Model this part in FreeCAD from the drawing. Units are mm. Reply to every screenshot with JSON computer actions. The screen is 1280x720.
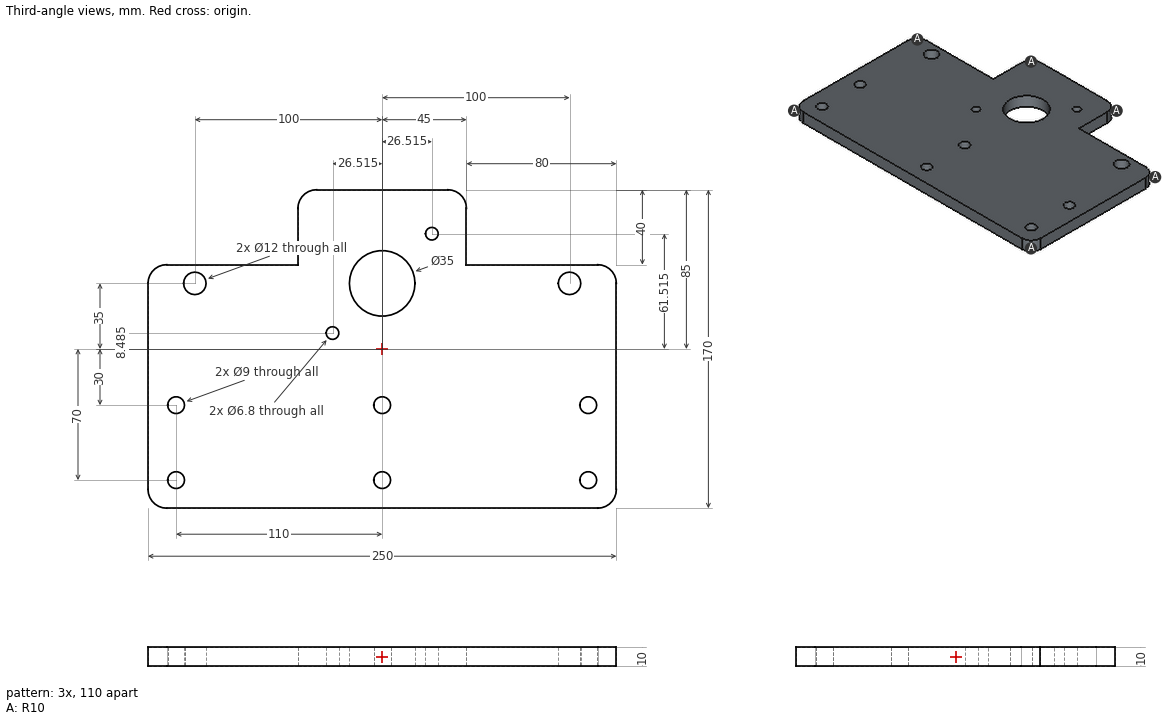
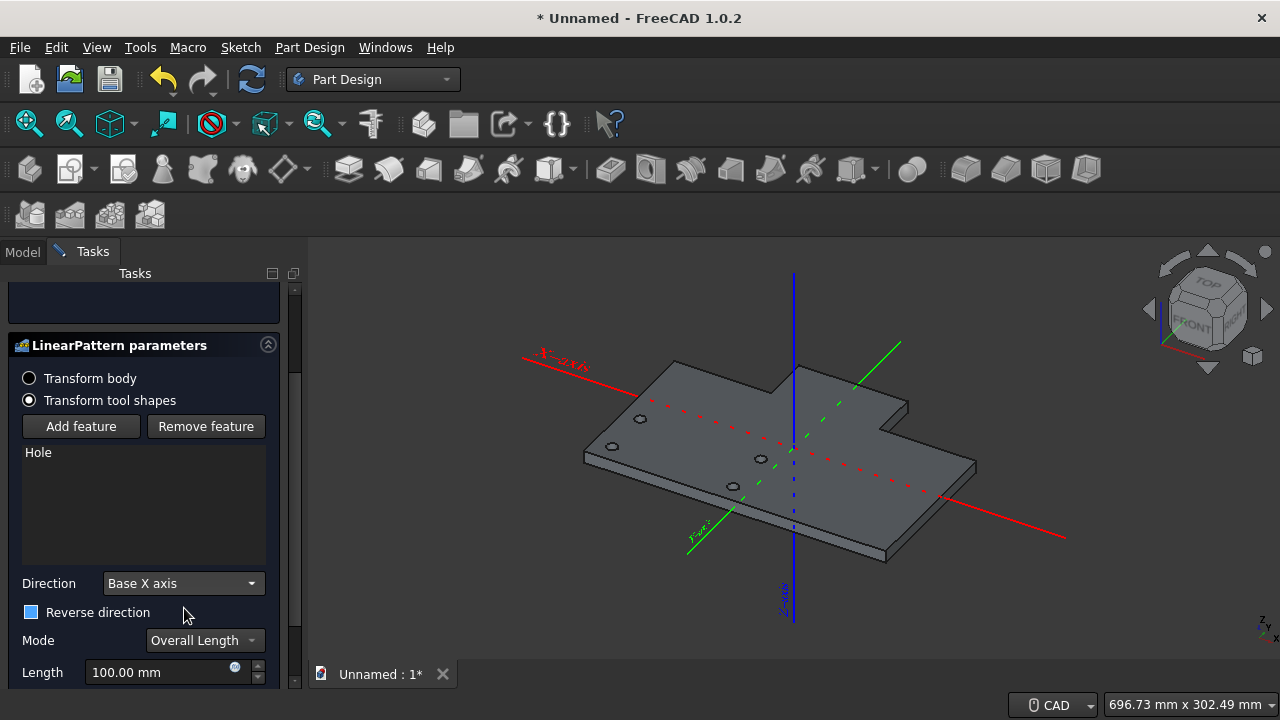
{"action": "left_click", "coordinate": [206, 640]}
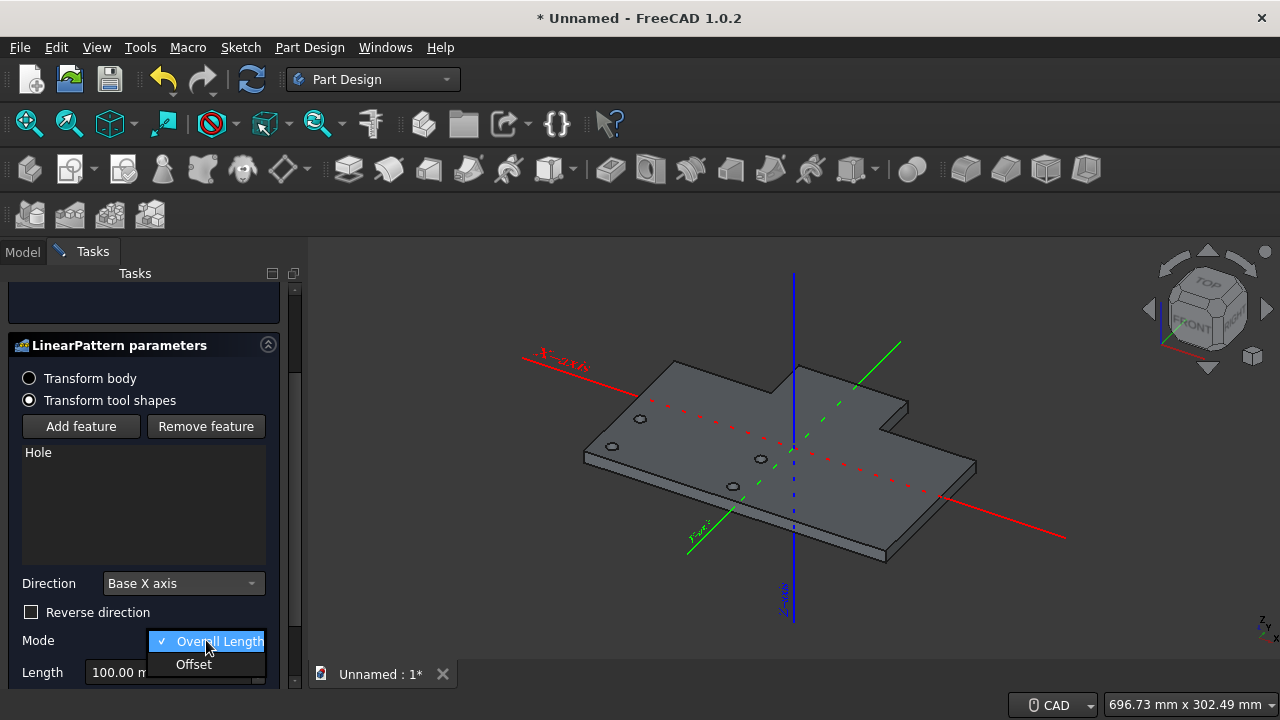
{"action": "left_click", "coordinate": [206, 664]}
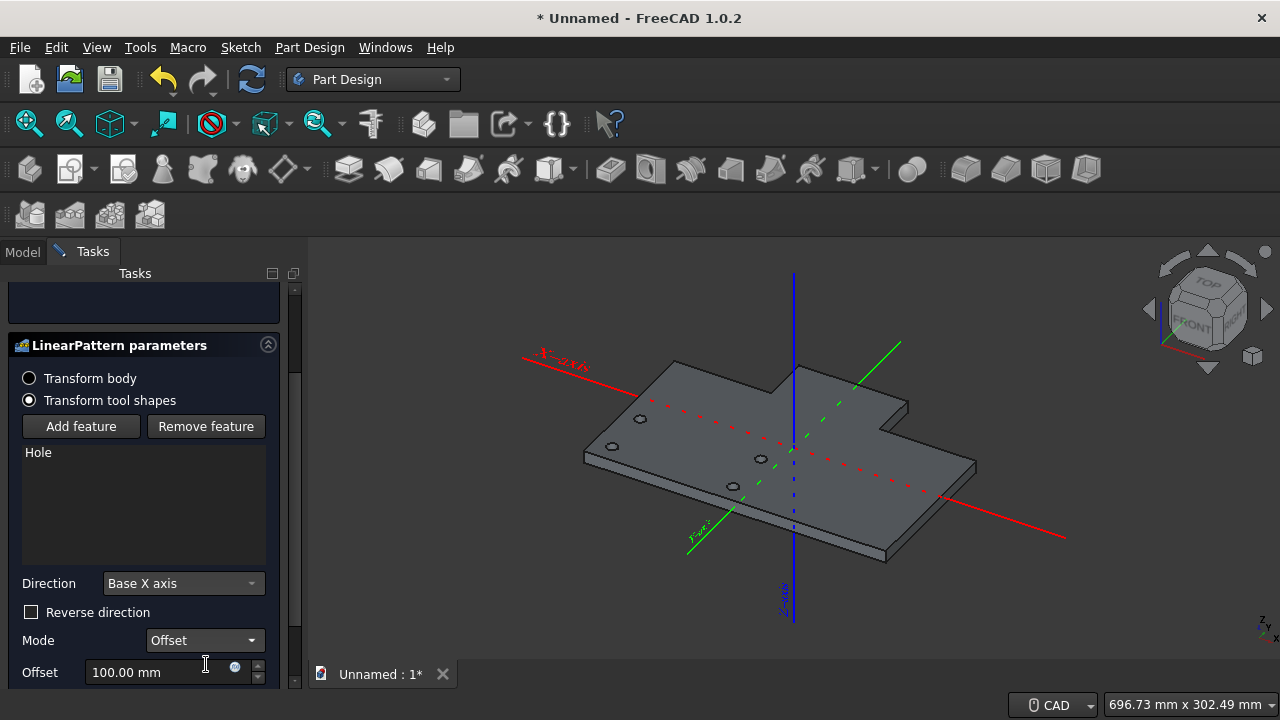
{"action": "triple_click", "coordinate": [168, 672]}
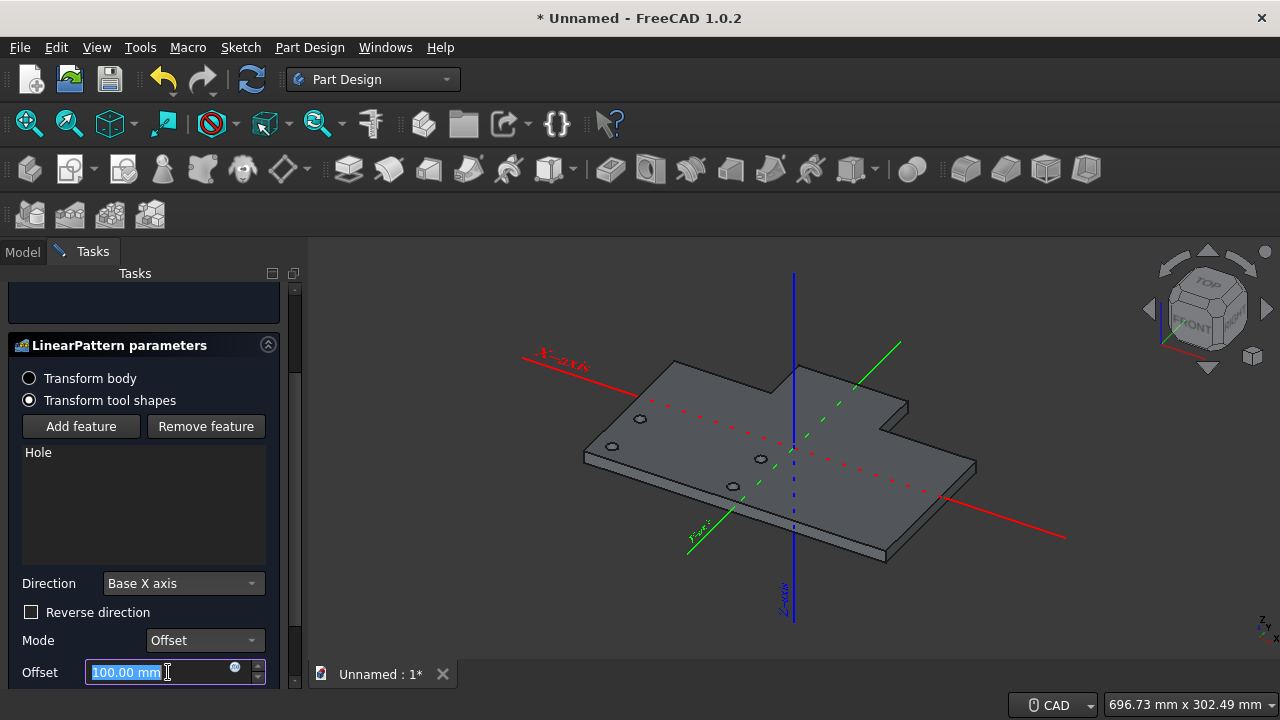
{"action": "type", "text": "110"}
{"action": "key", "text": "Tab"}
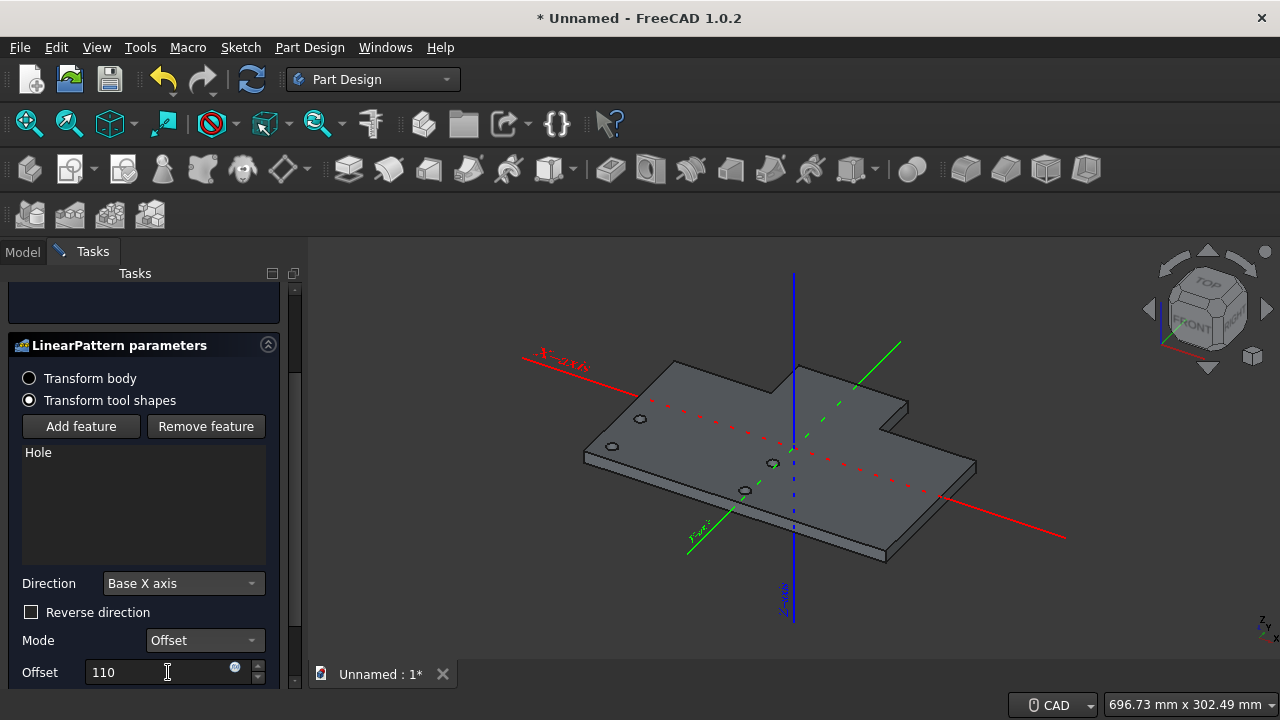
{"action": "scroll", "coordinate": [295, 486], "scroll_direction": "down", "scroll_amount": 2}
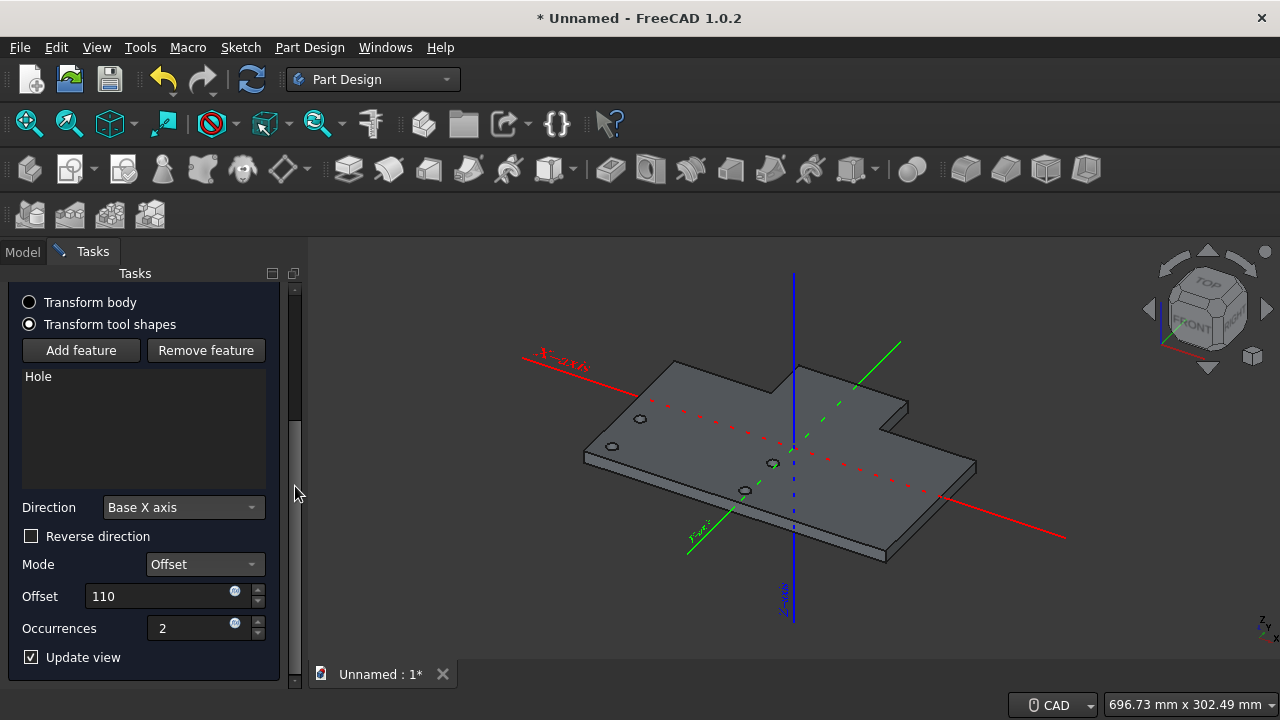
{"action": "triple_click", "coordinate": [198, 628]}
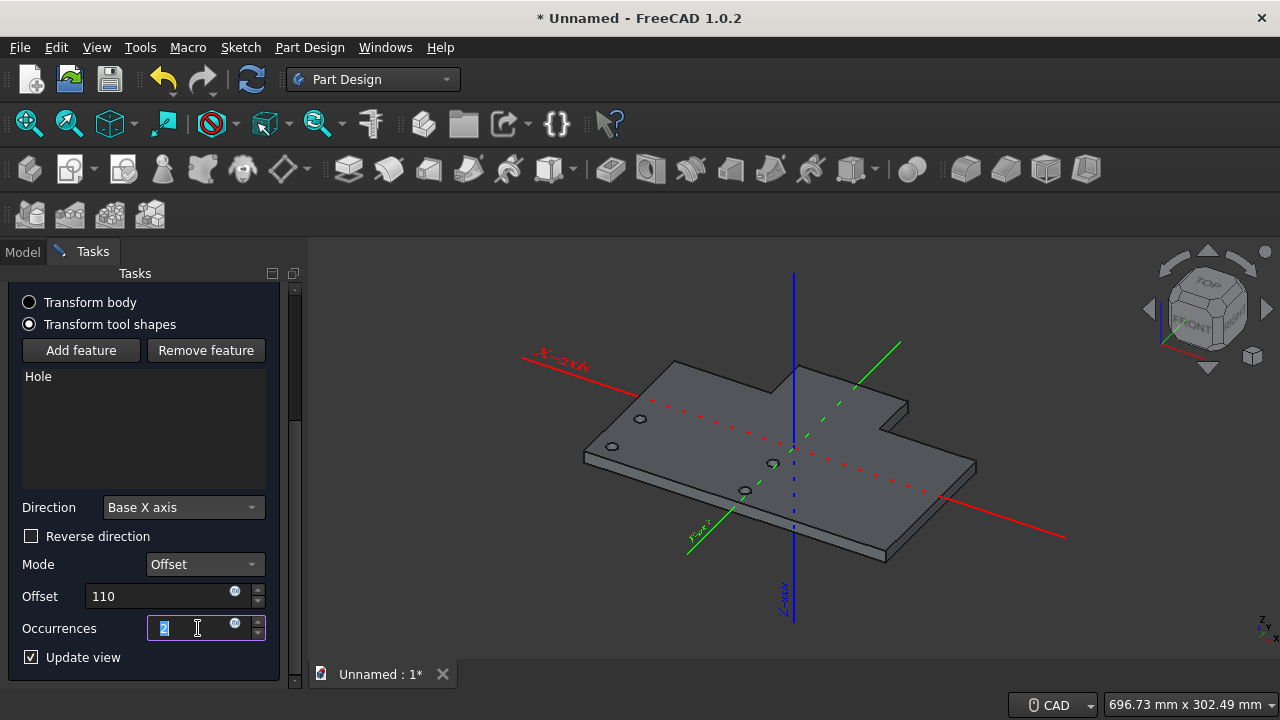
{"action": "type", "text": "3"}
{"action": "key", "text": "Tab"}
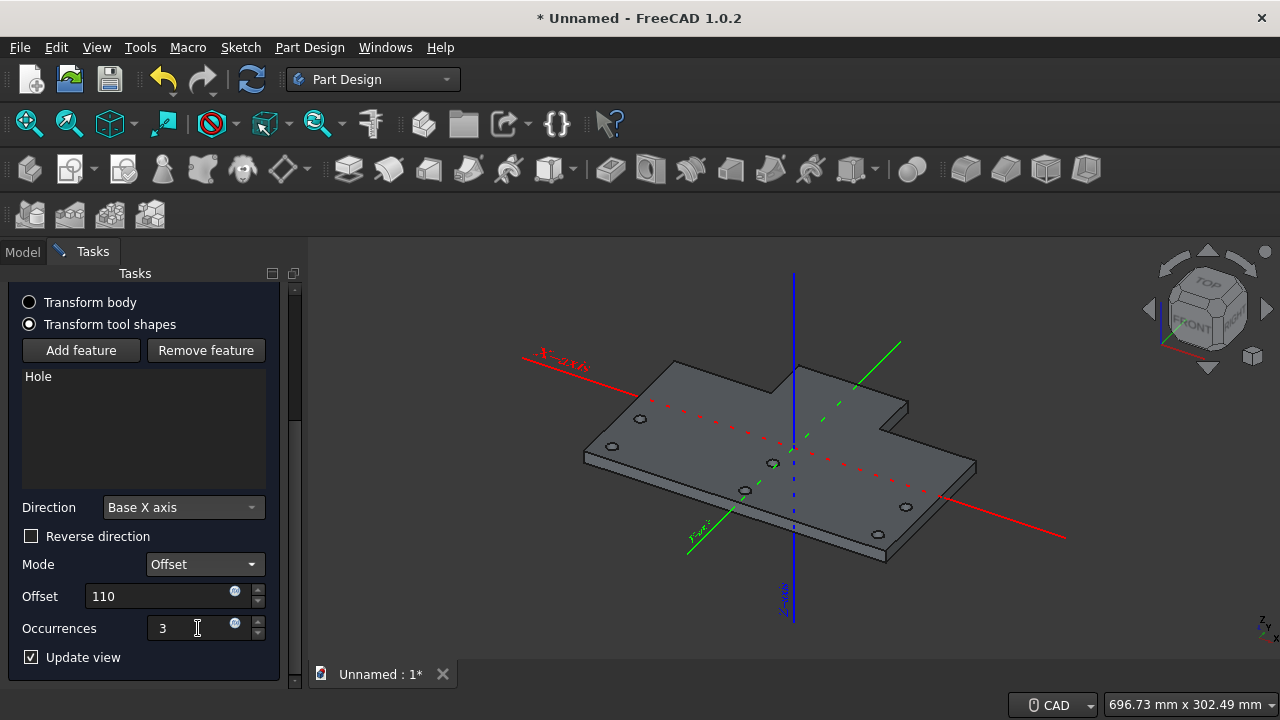
{"action": "scroll", "coordinate": [295, 486], "scroll_direction": "up", "scroll_amount": 5}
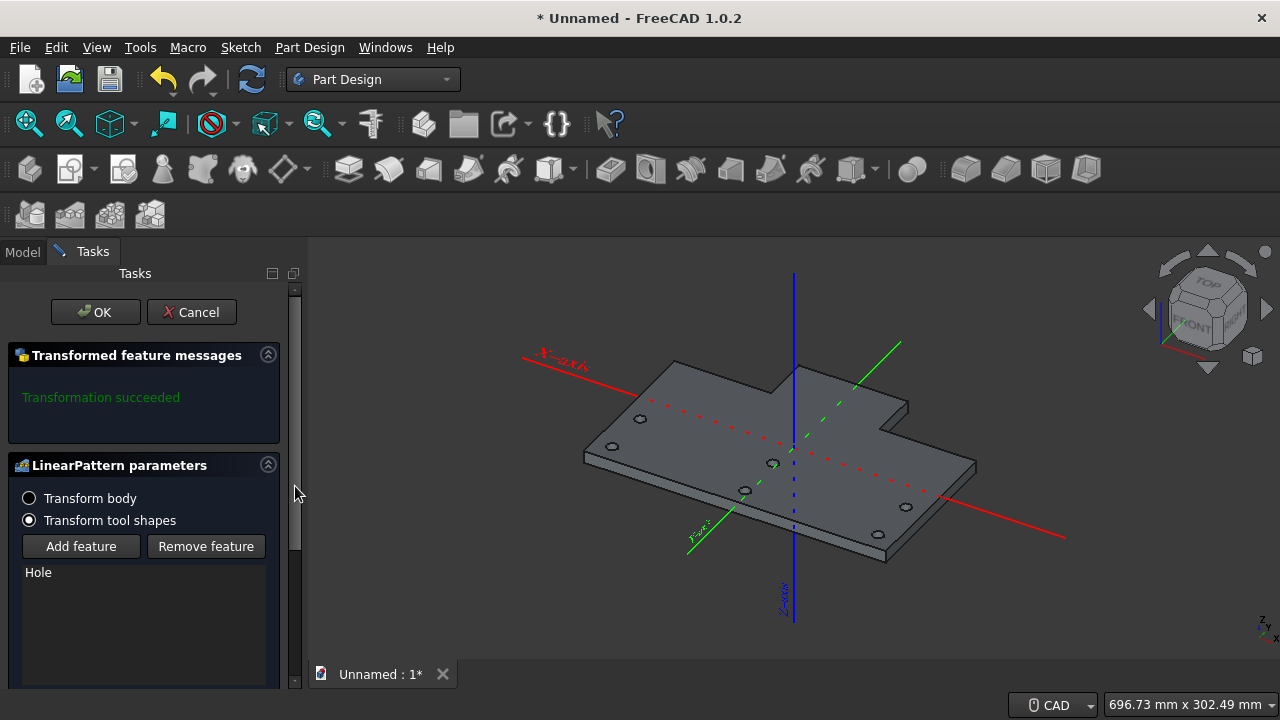
{"action": "left_click", "coordinate": [96, 312]}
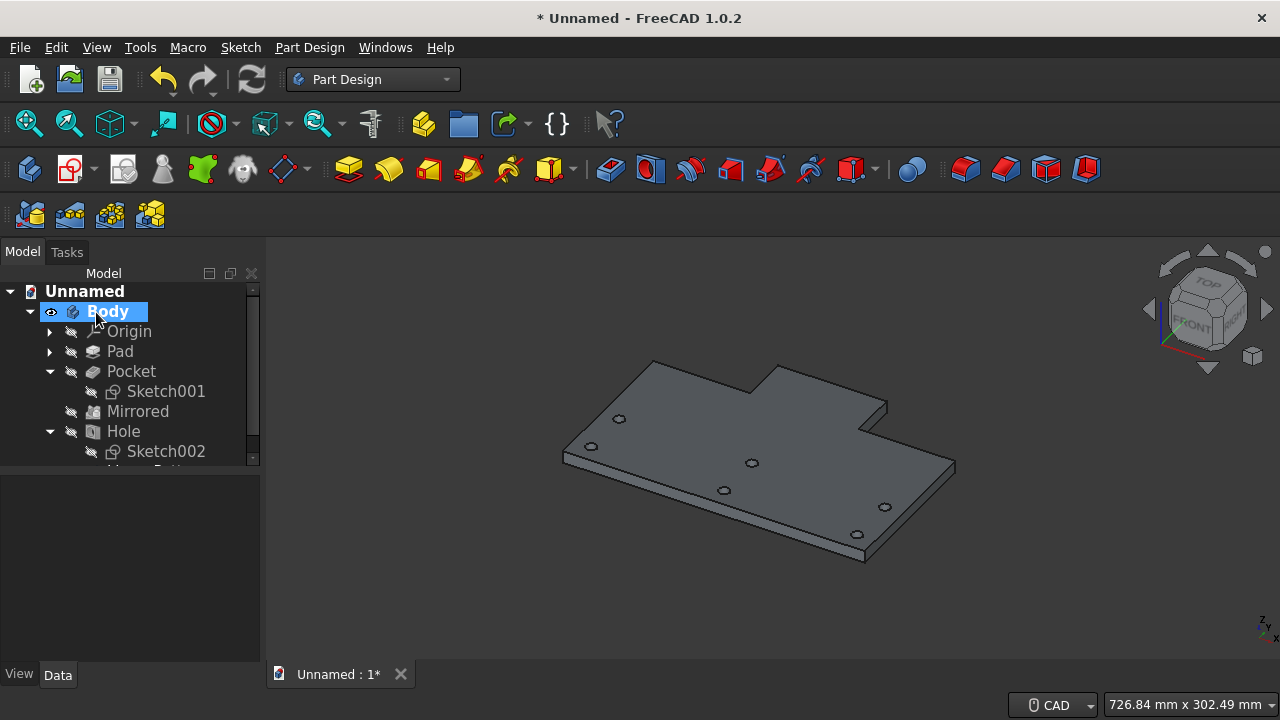
{"action": "left_click", "coordinate": [790, 424]}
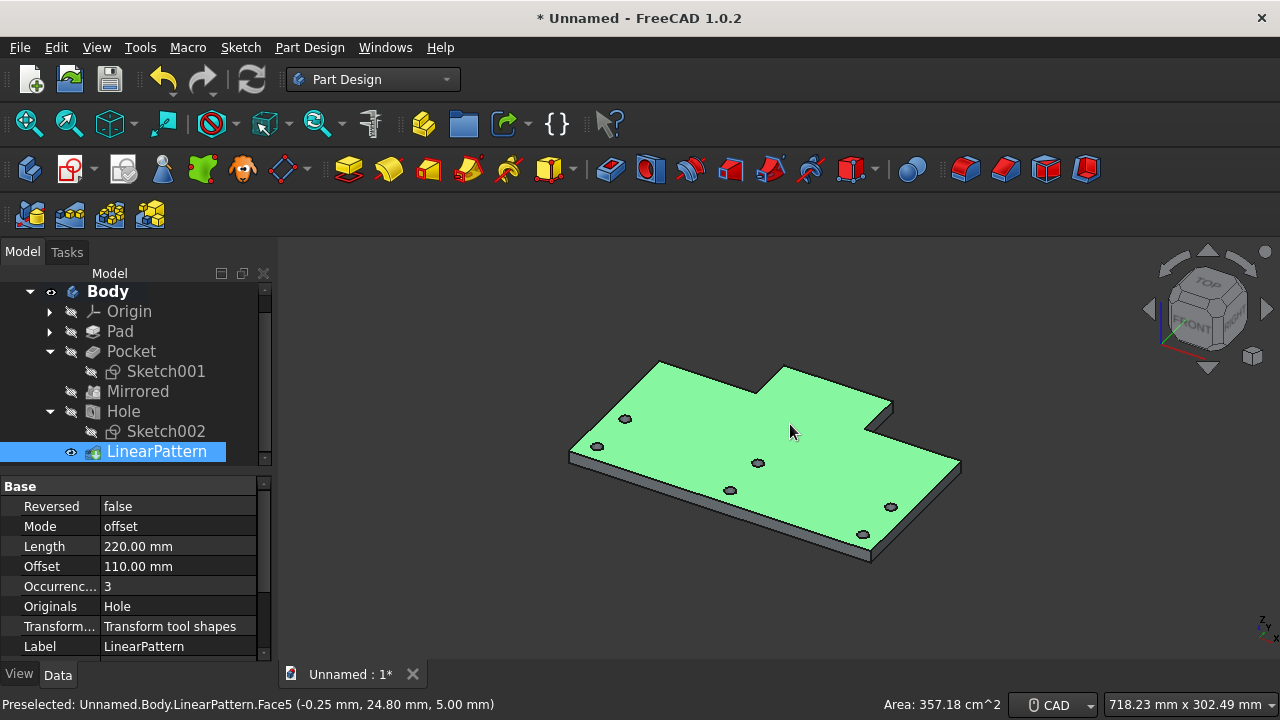
{"action": "left_click", "coordinate": [70, 170]}